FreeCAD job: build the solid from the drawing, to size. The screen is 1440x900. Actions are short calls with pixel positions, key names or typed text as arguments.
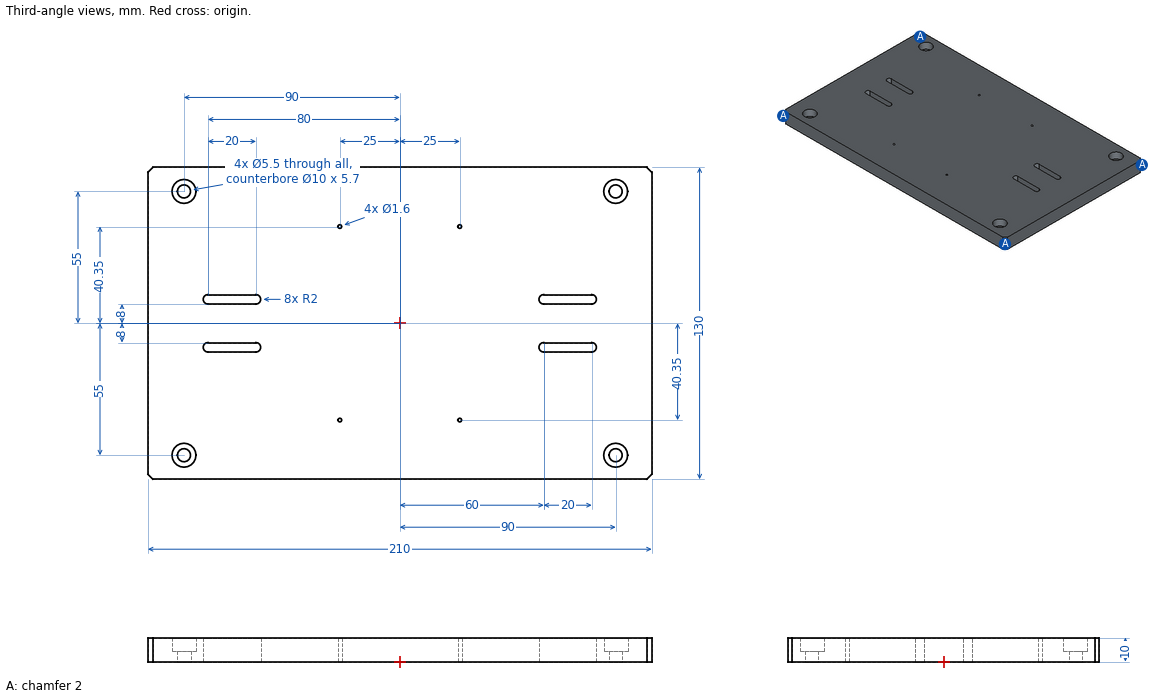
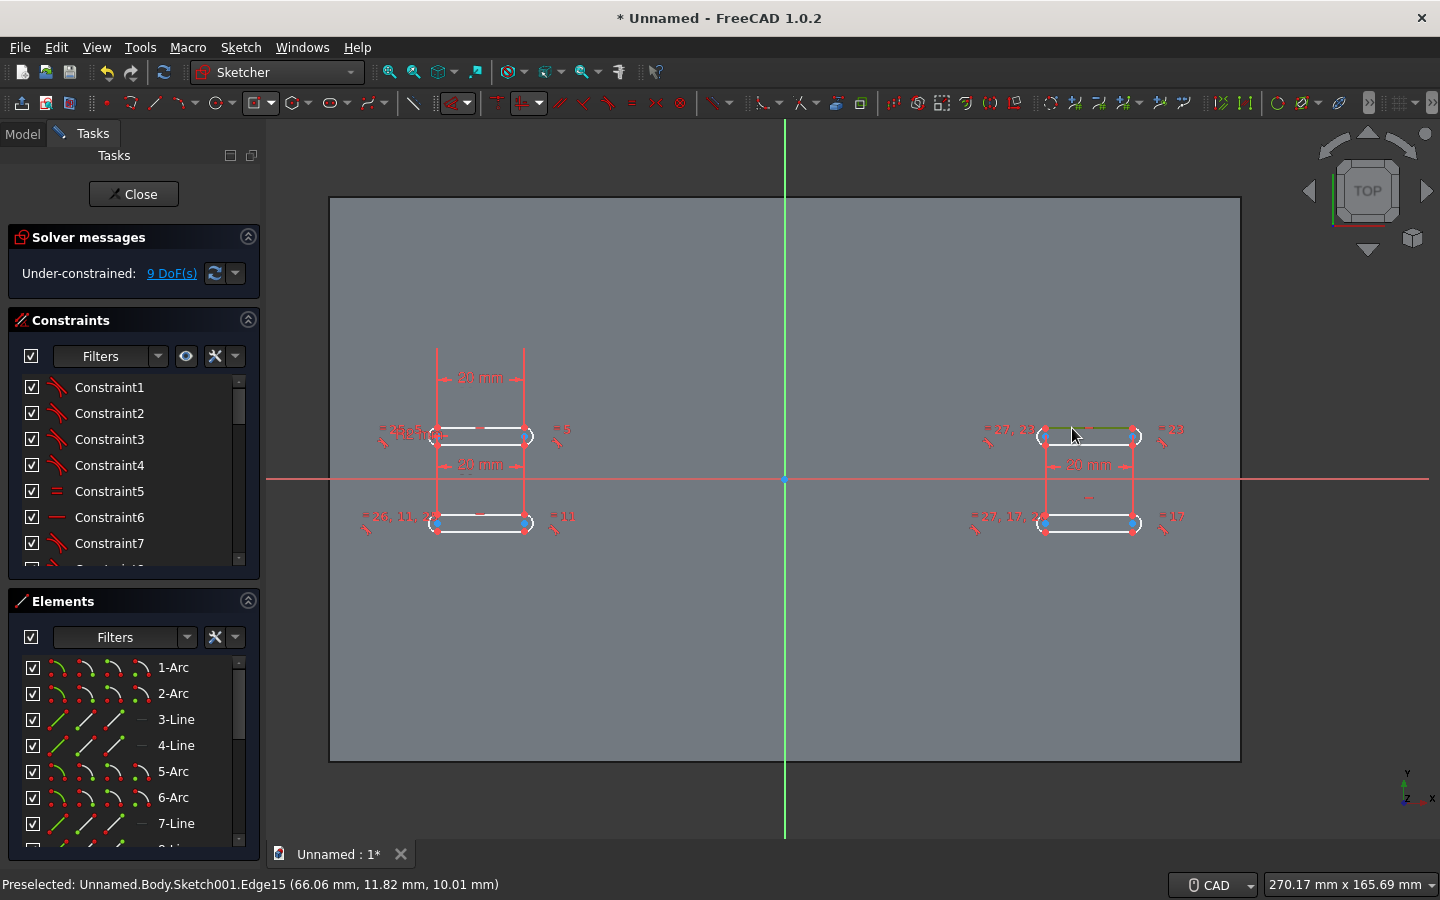
key(l)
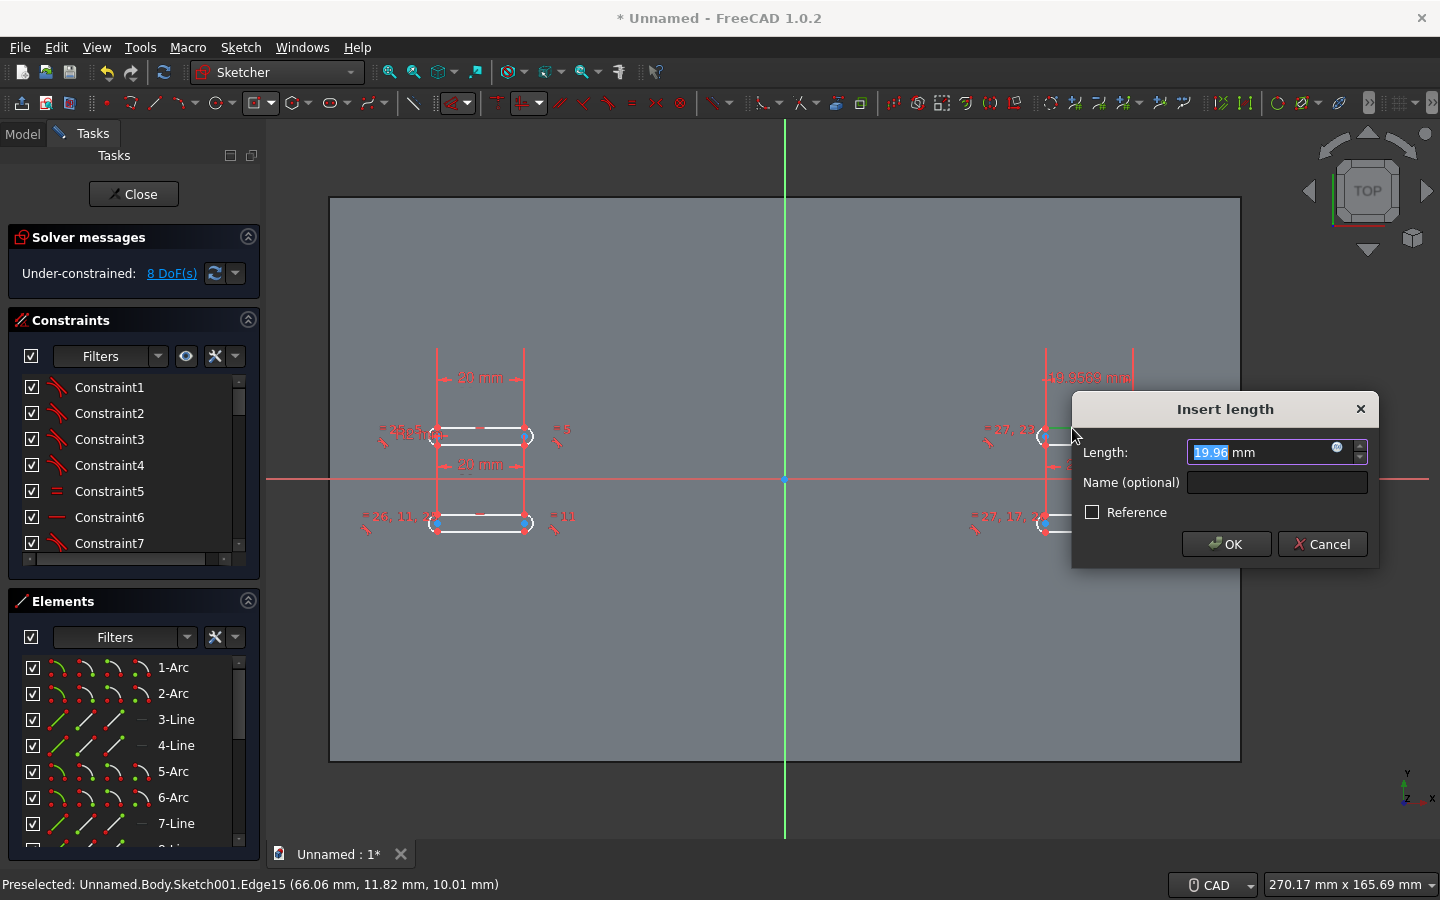
text(20)
key(Return)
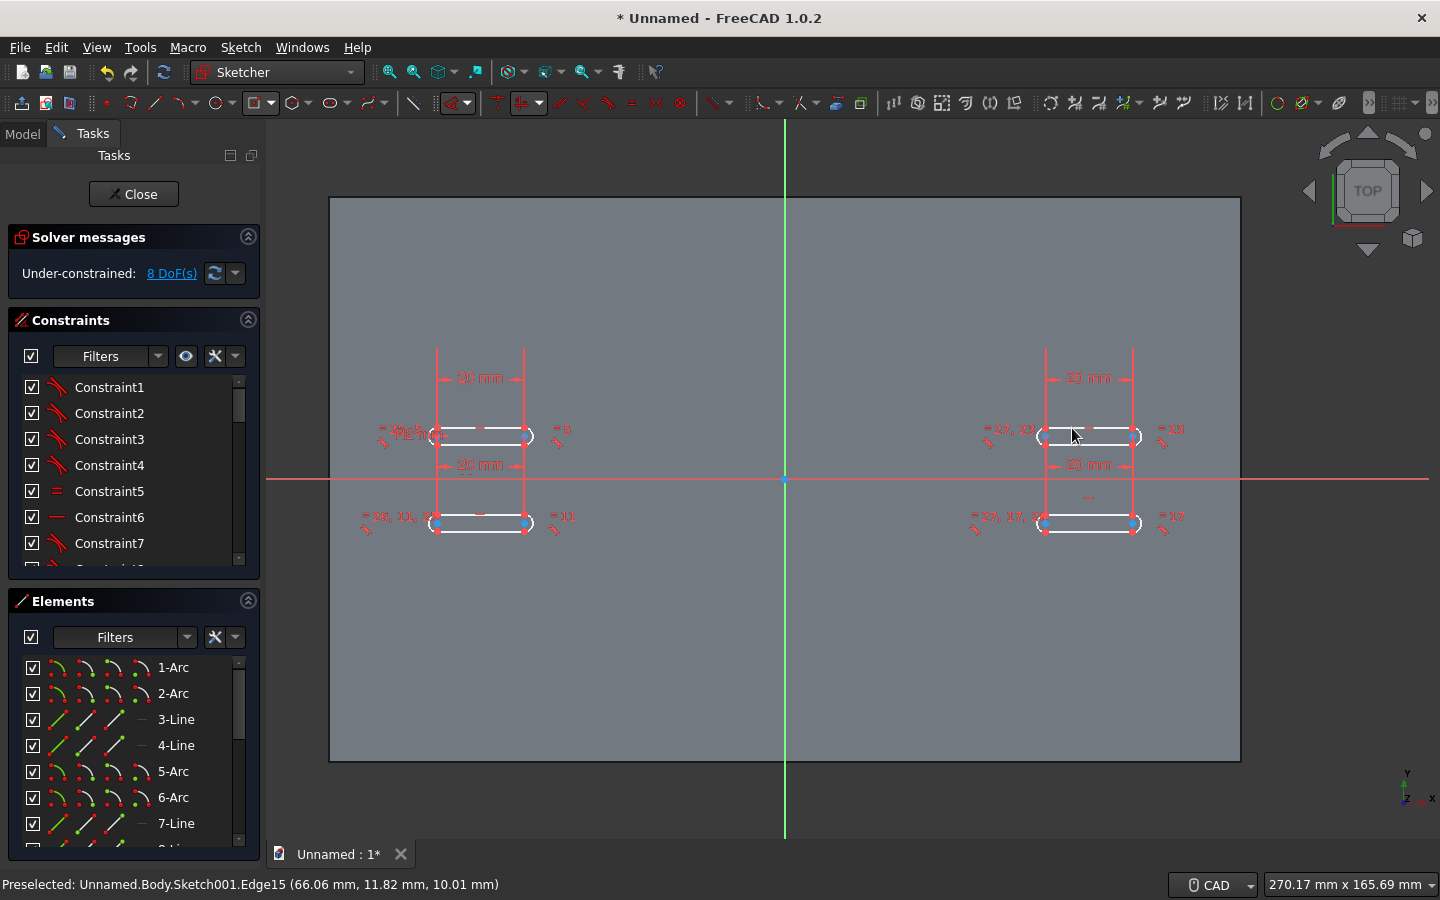
scroll(437, 445, up, 2)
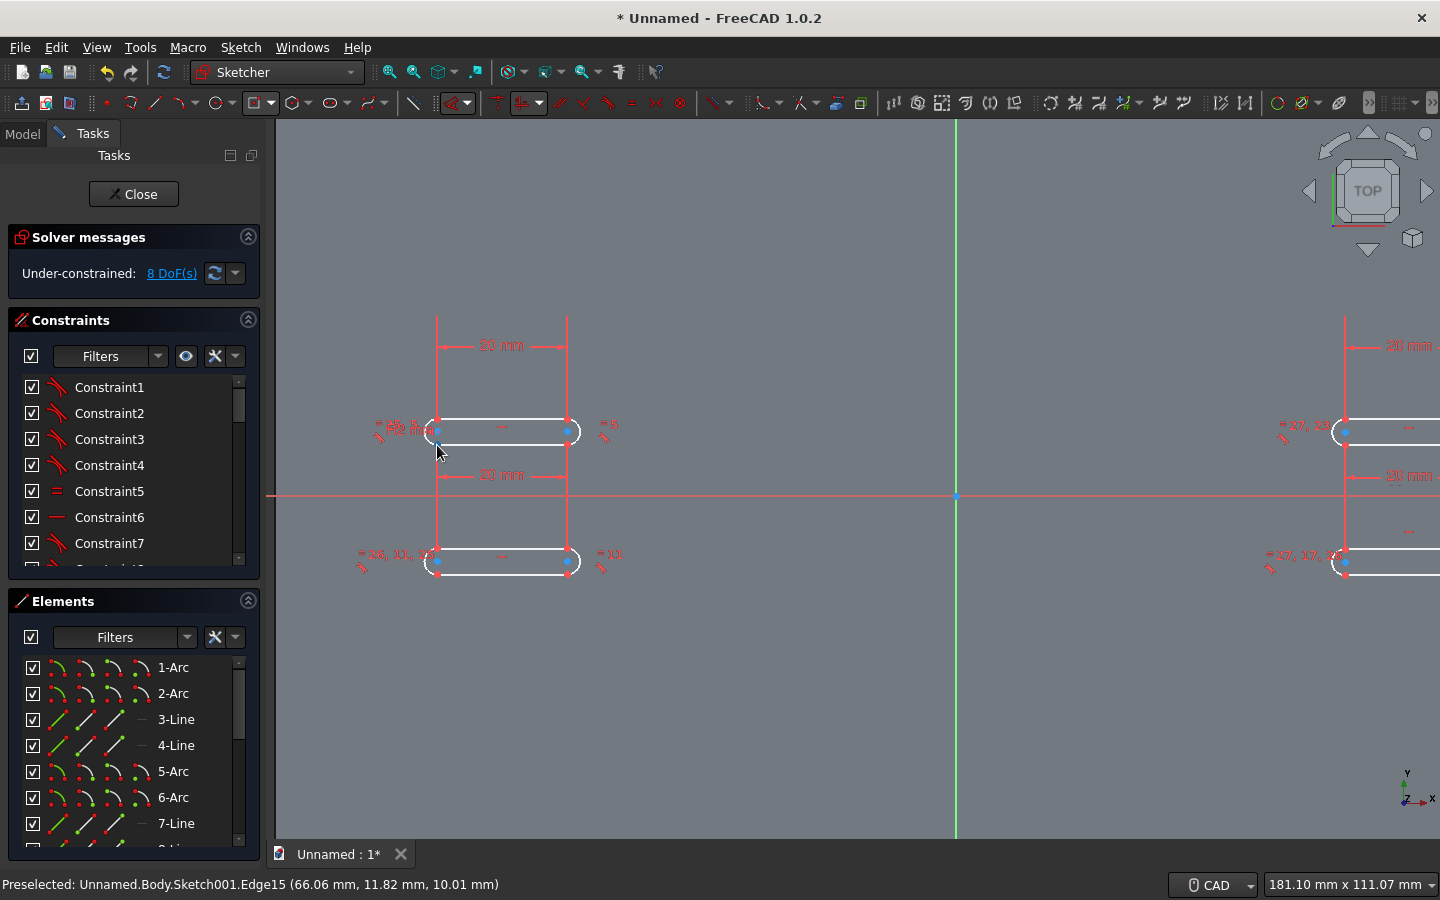
click(437, 445)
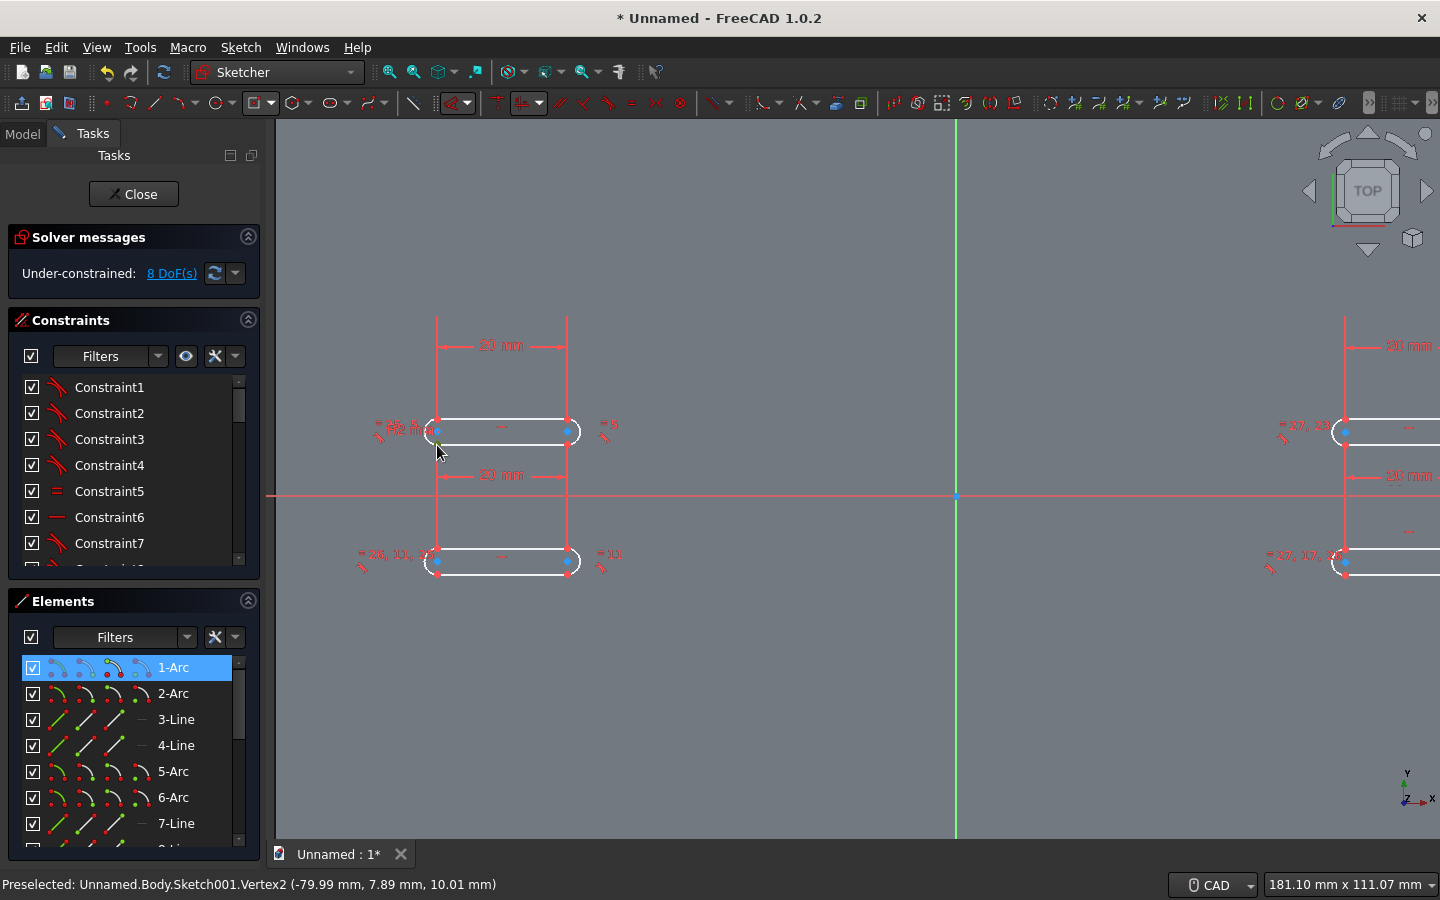
click(470, 104)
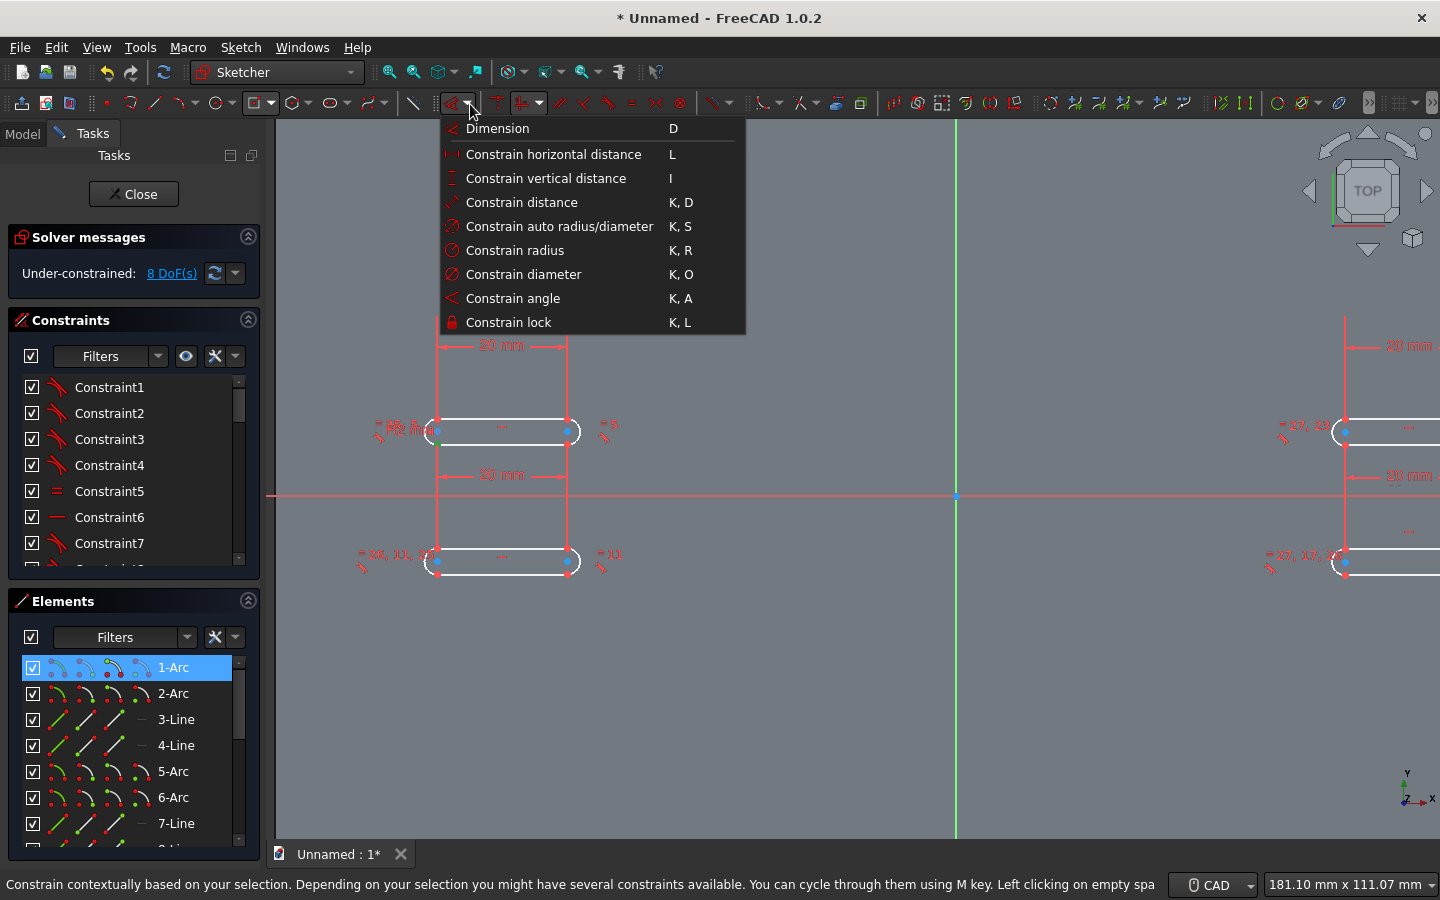
click(593, 178)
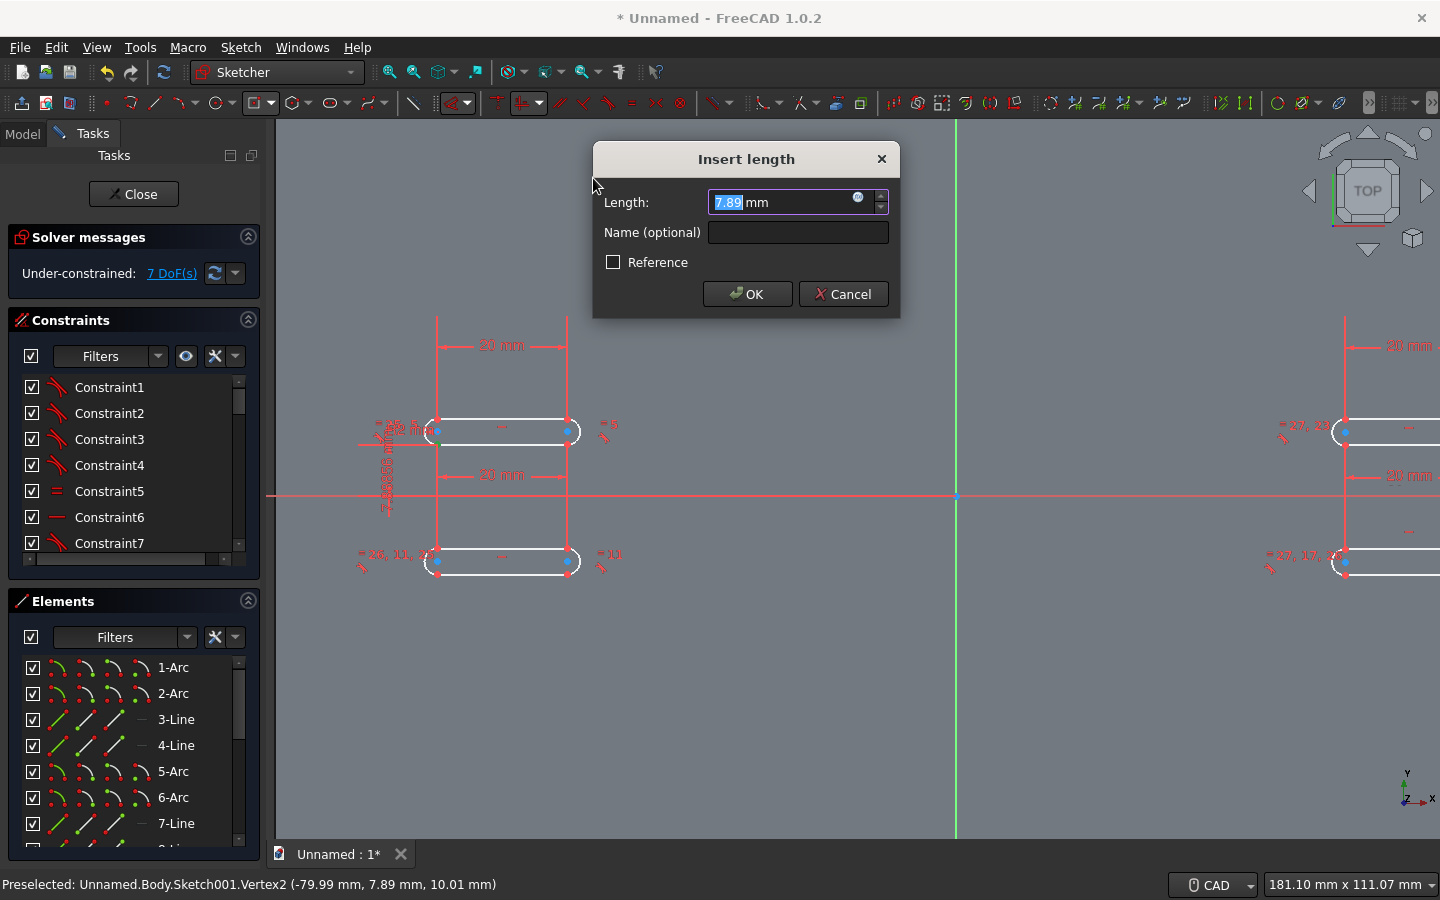
text(8)
key(Return)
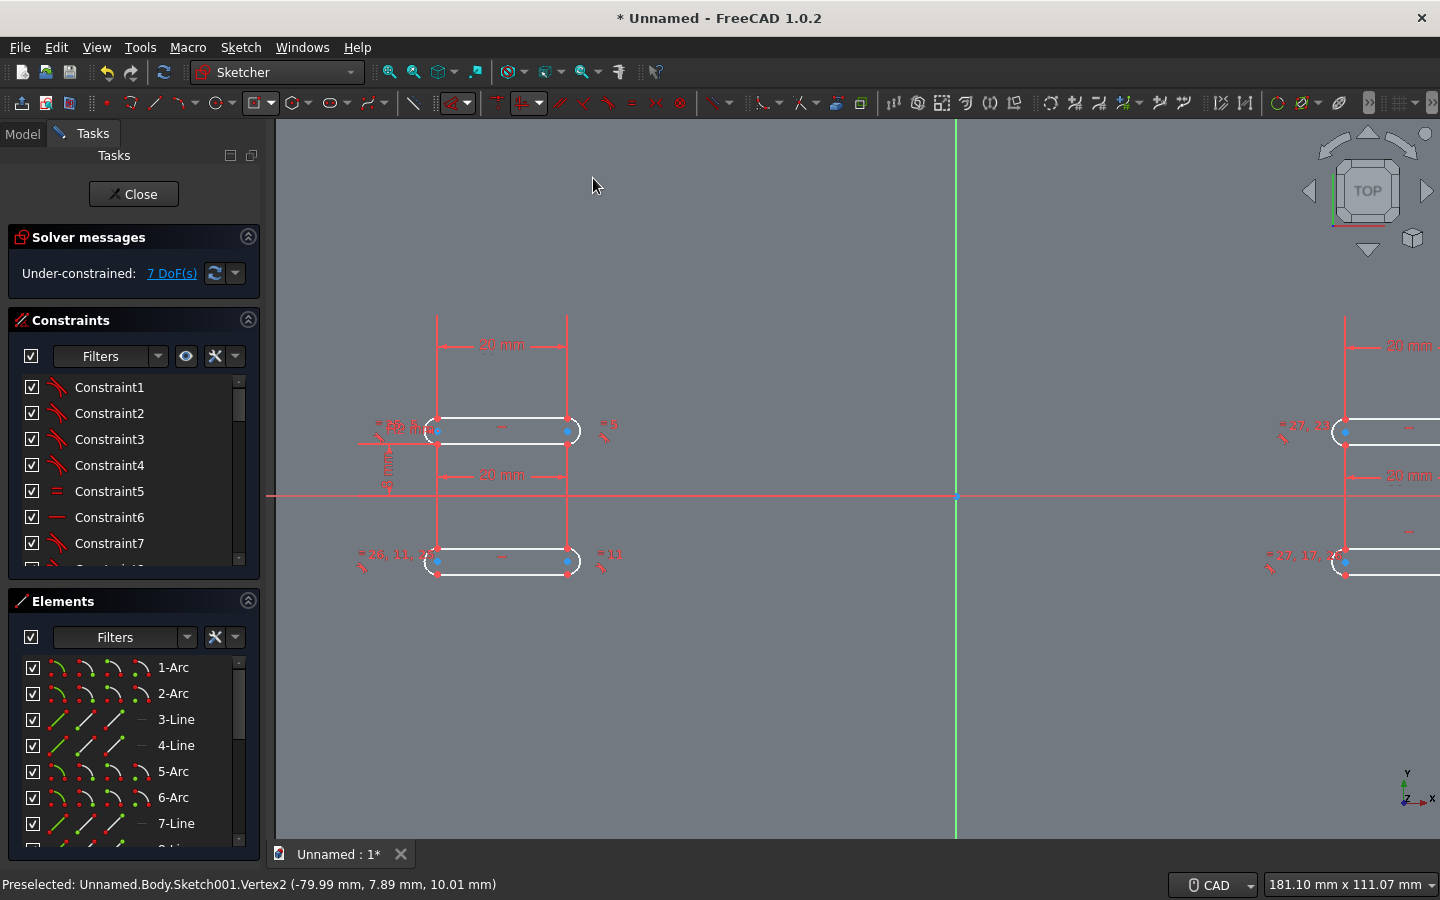
click(437, 549)